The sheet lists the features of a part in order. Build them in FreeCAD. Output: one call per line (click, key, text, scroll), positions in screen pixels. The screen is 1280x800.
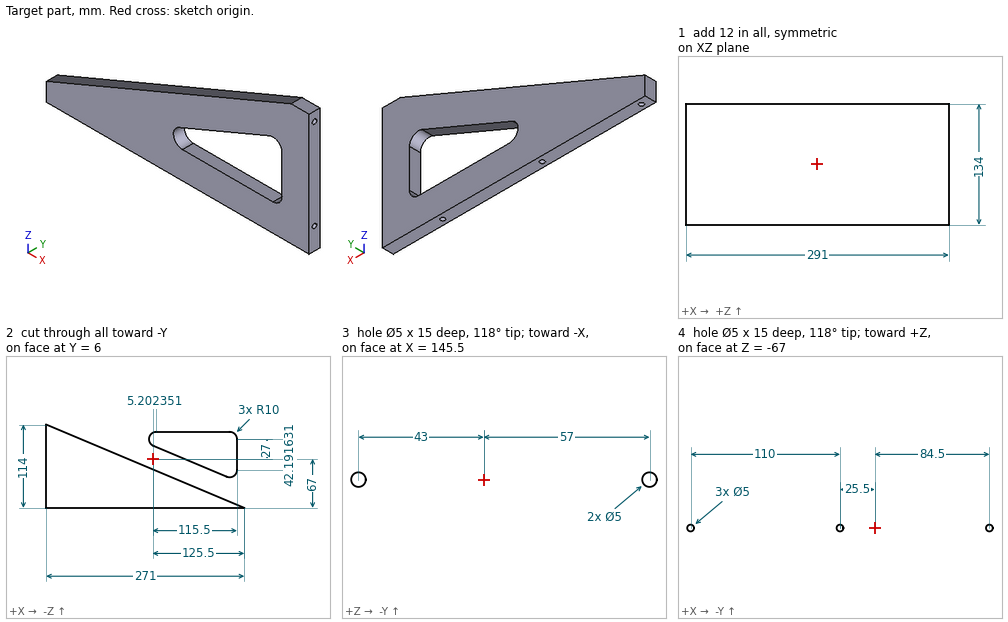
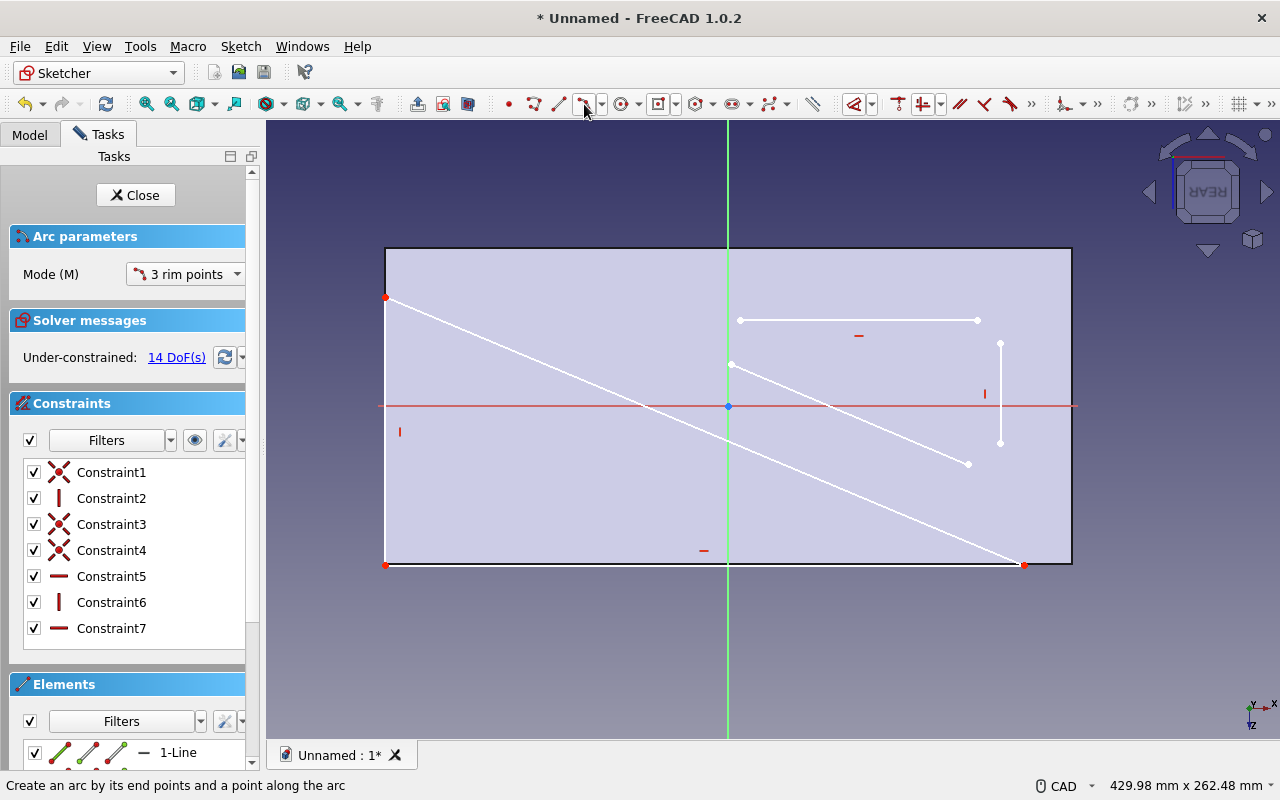
click(1001, 343)
click(978, 320)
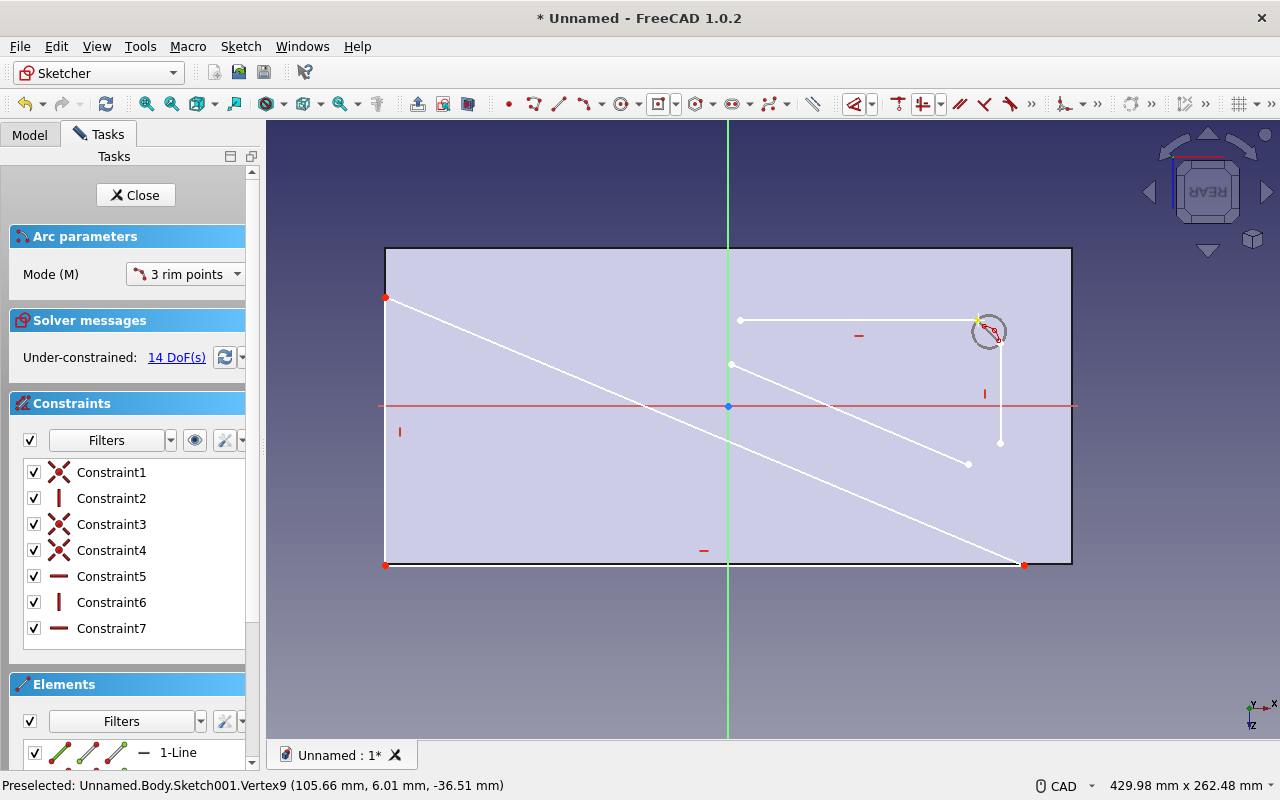
scroll(994, 326, up, 5)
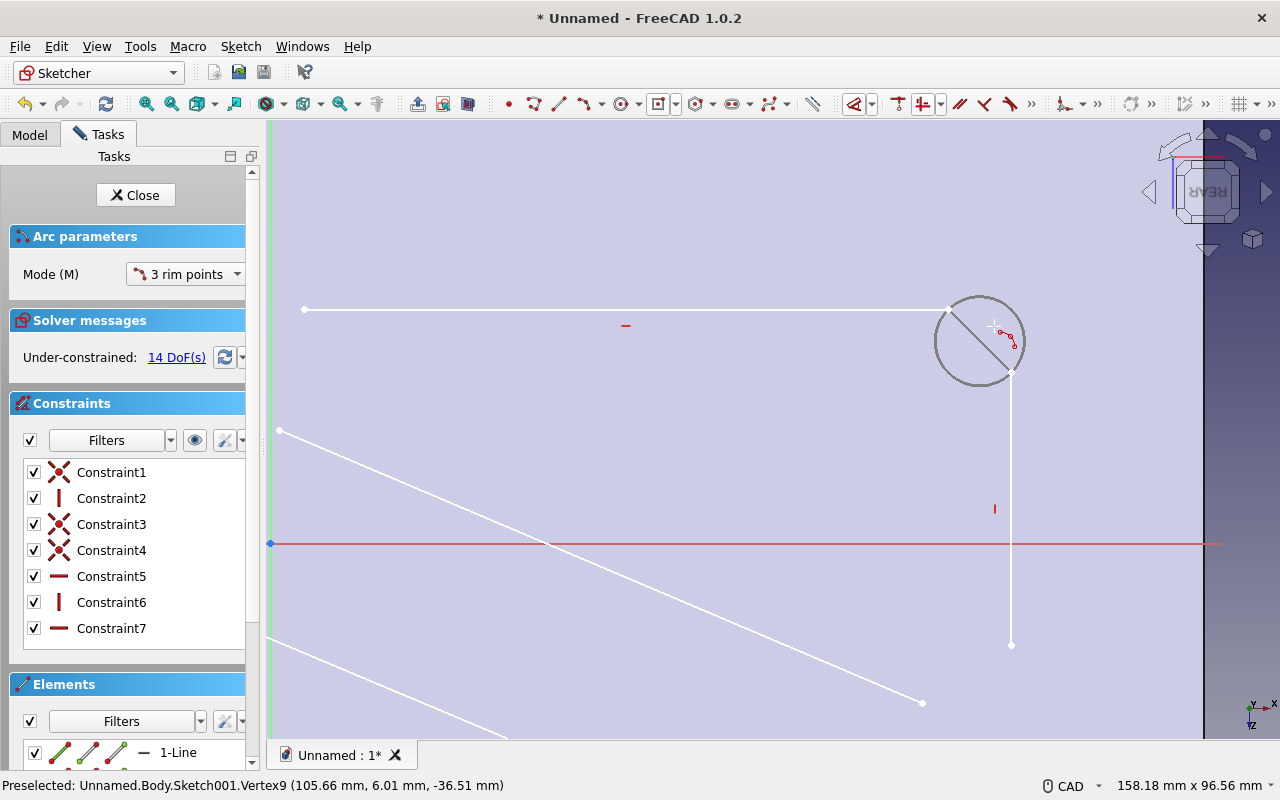
click(993, 325)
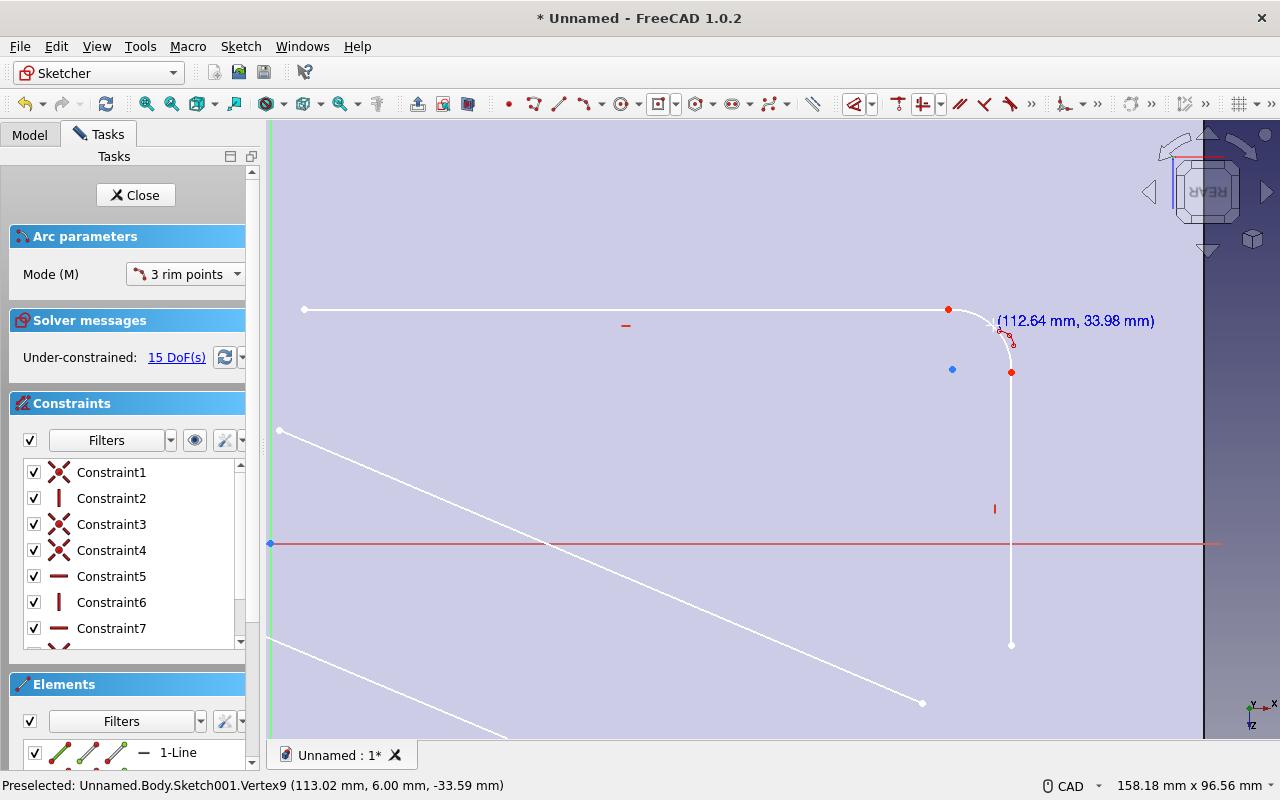
click(305, 310)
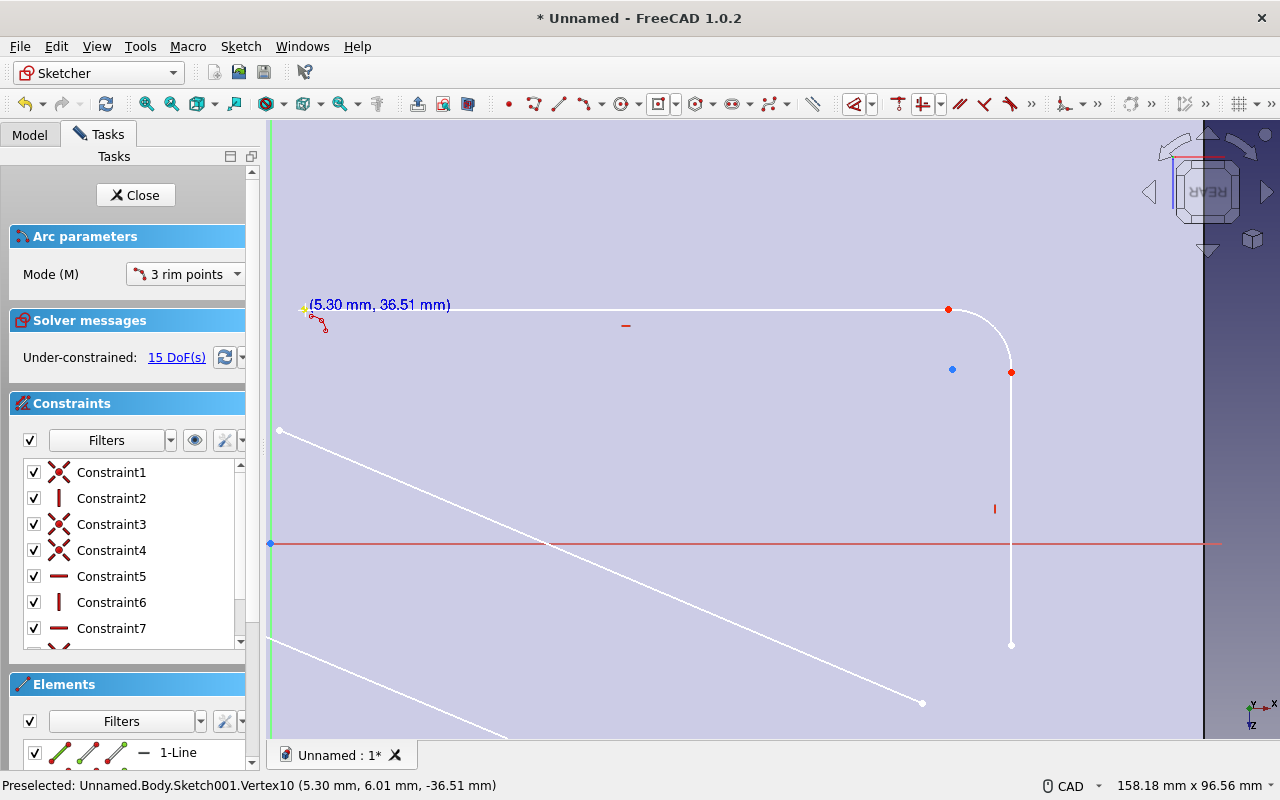
scroll(994, 326, down, 5)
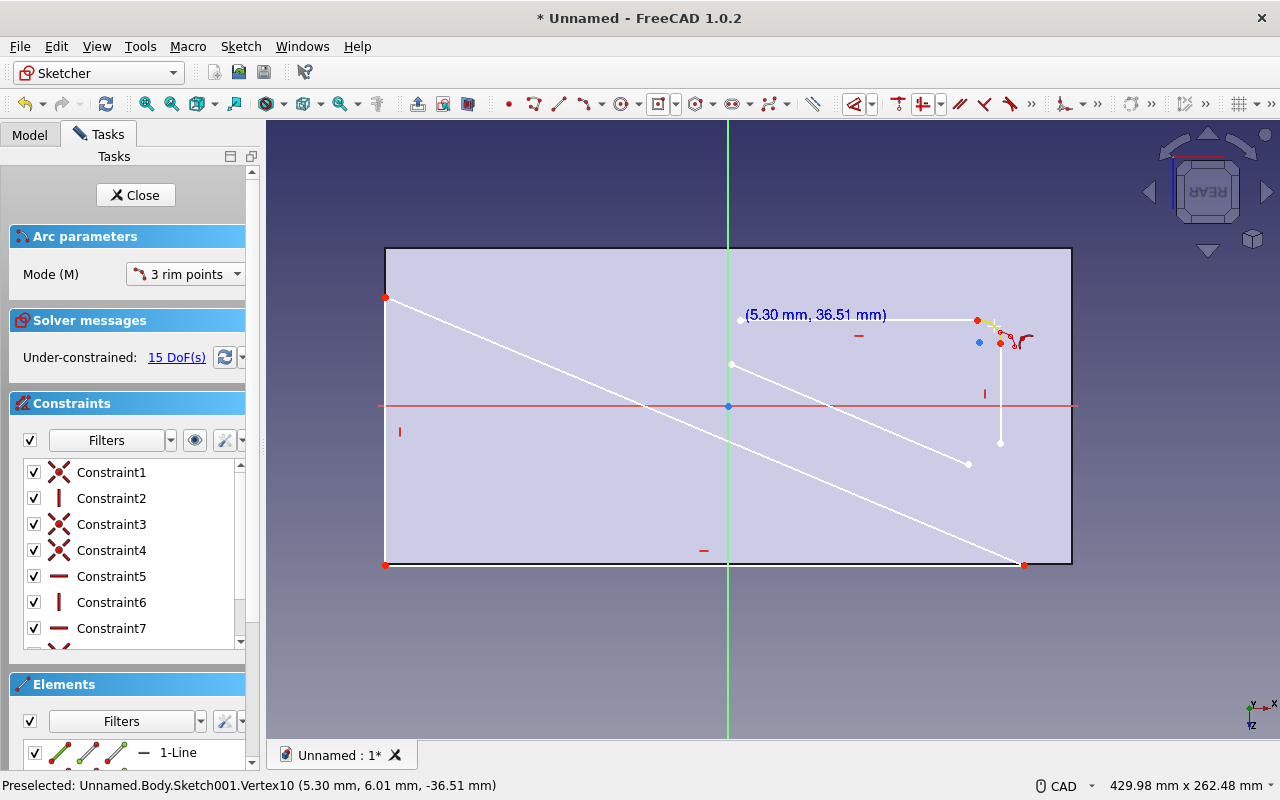
scroll(732, 364, up, 9)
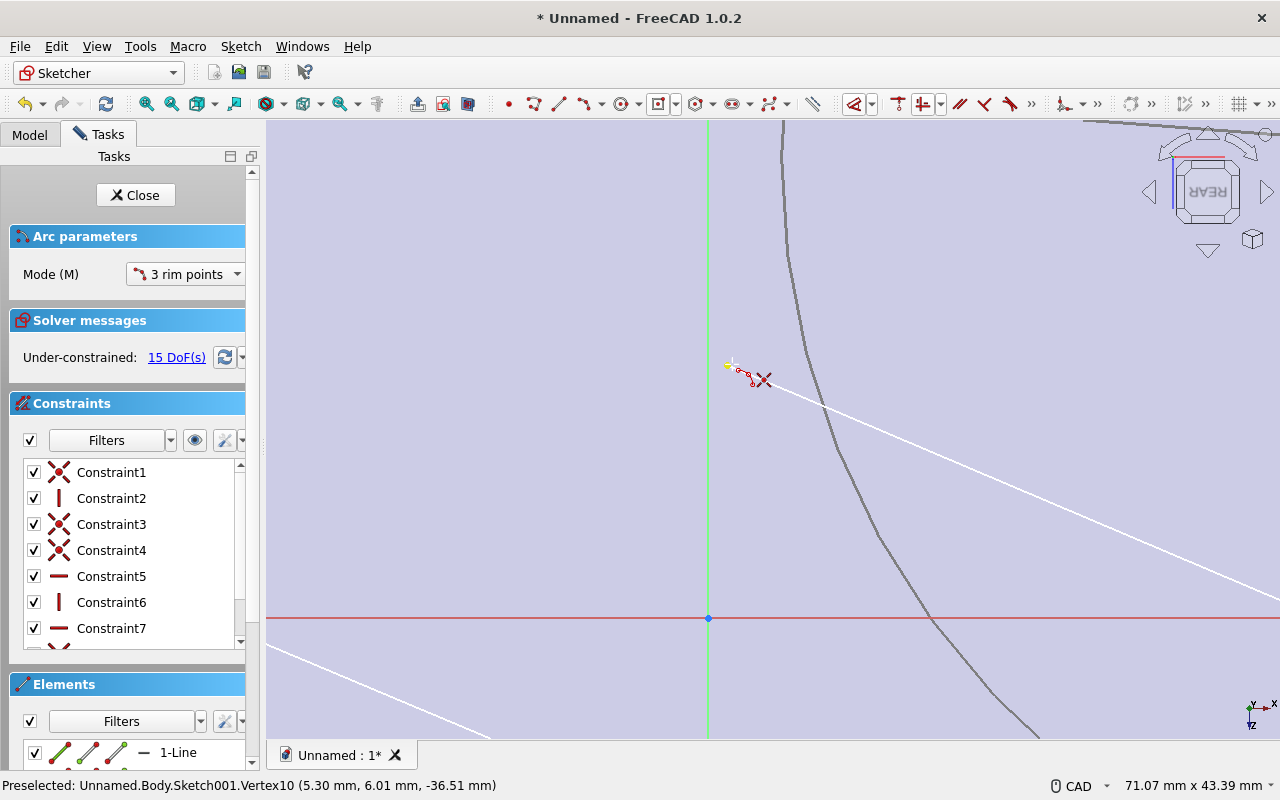
click(728, 365)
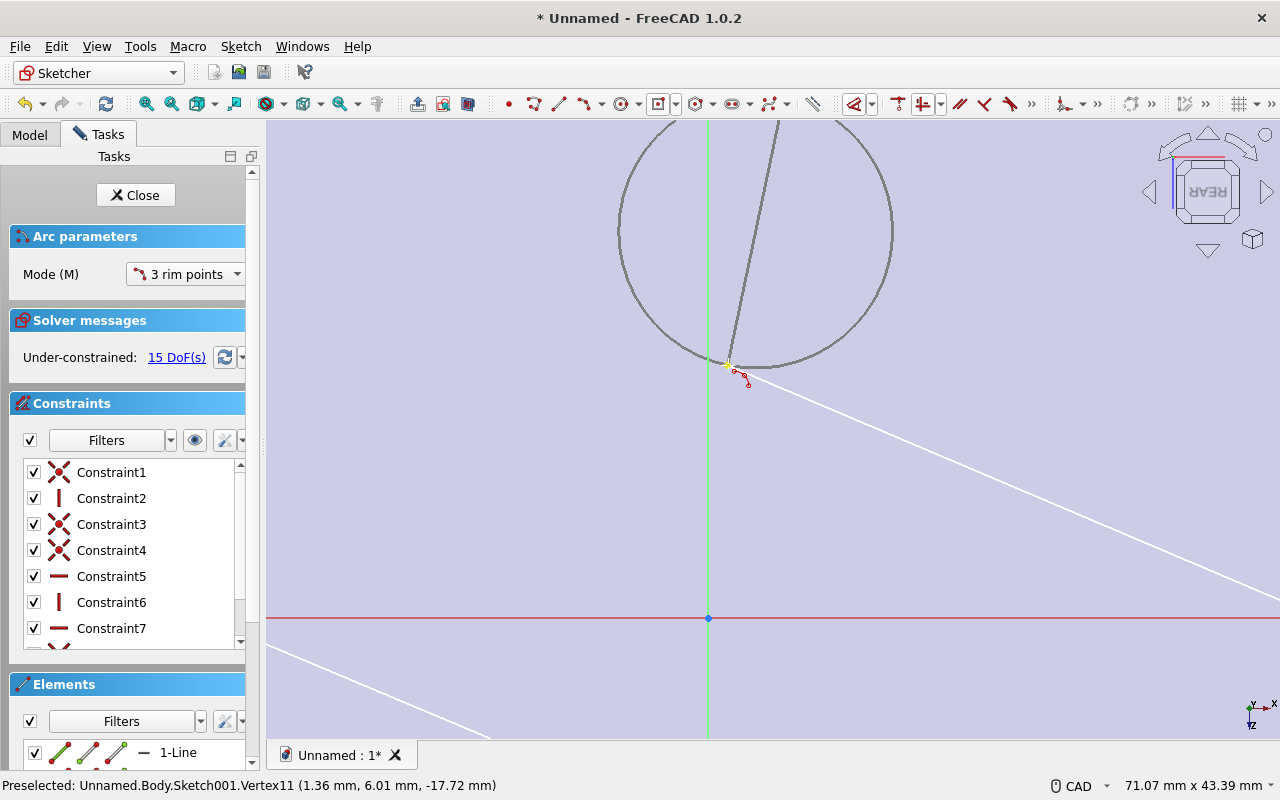
scroll(732, 364, down, 9)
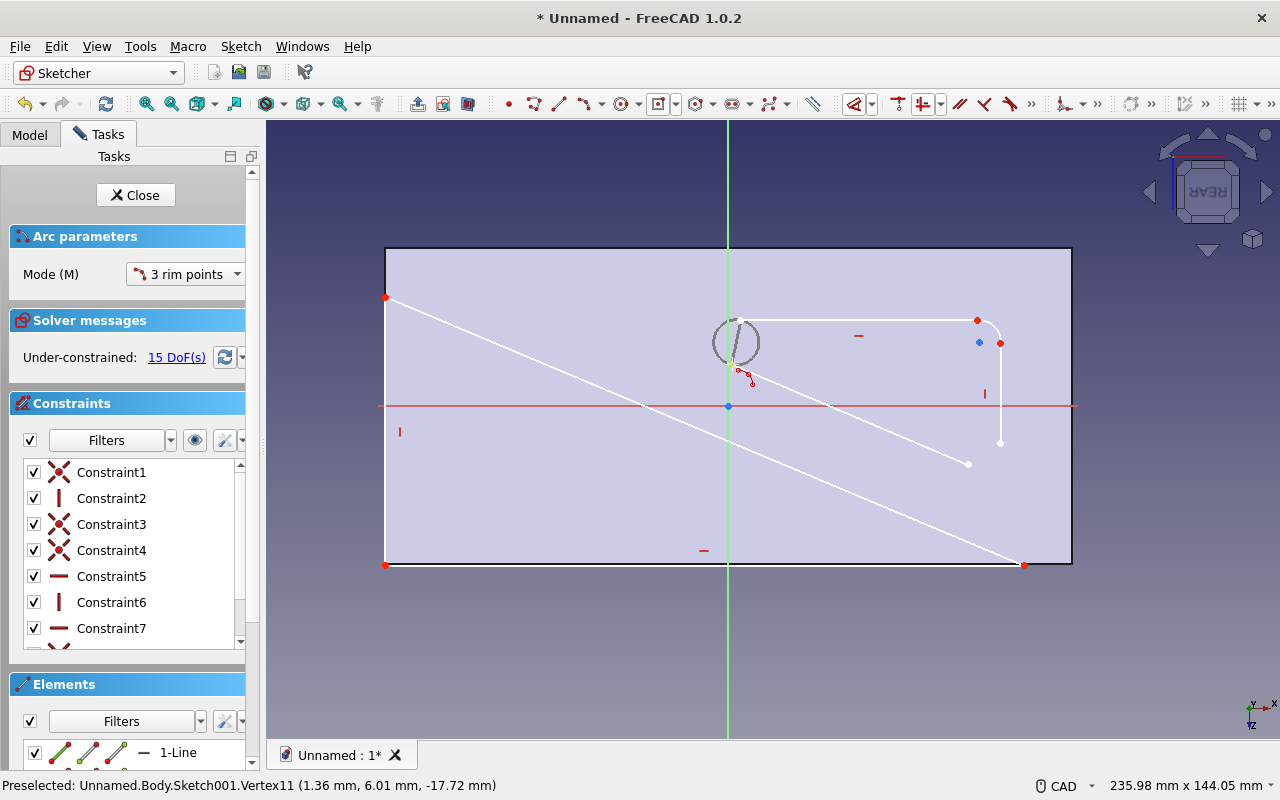
scroll(717, 344, up, 2)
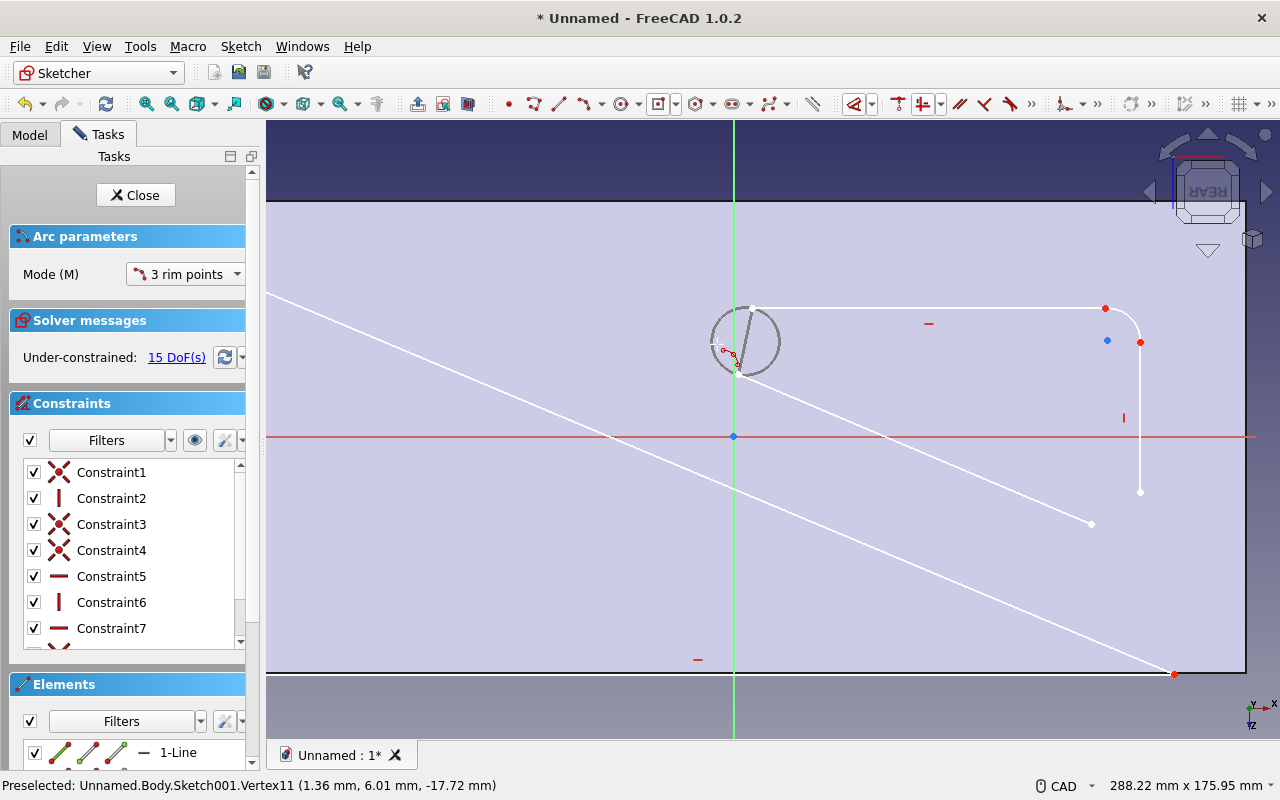
click(717, 344)